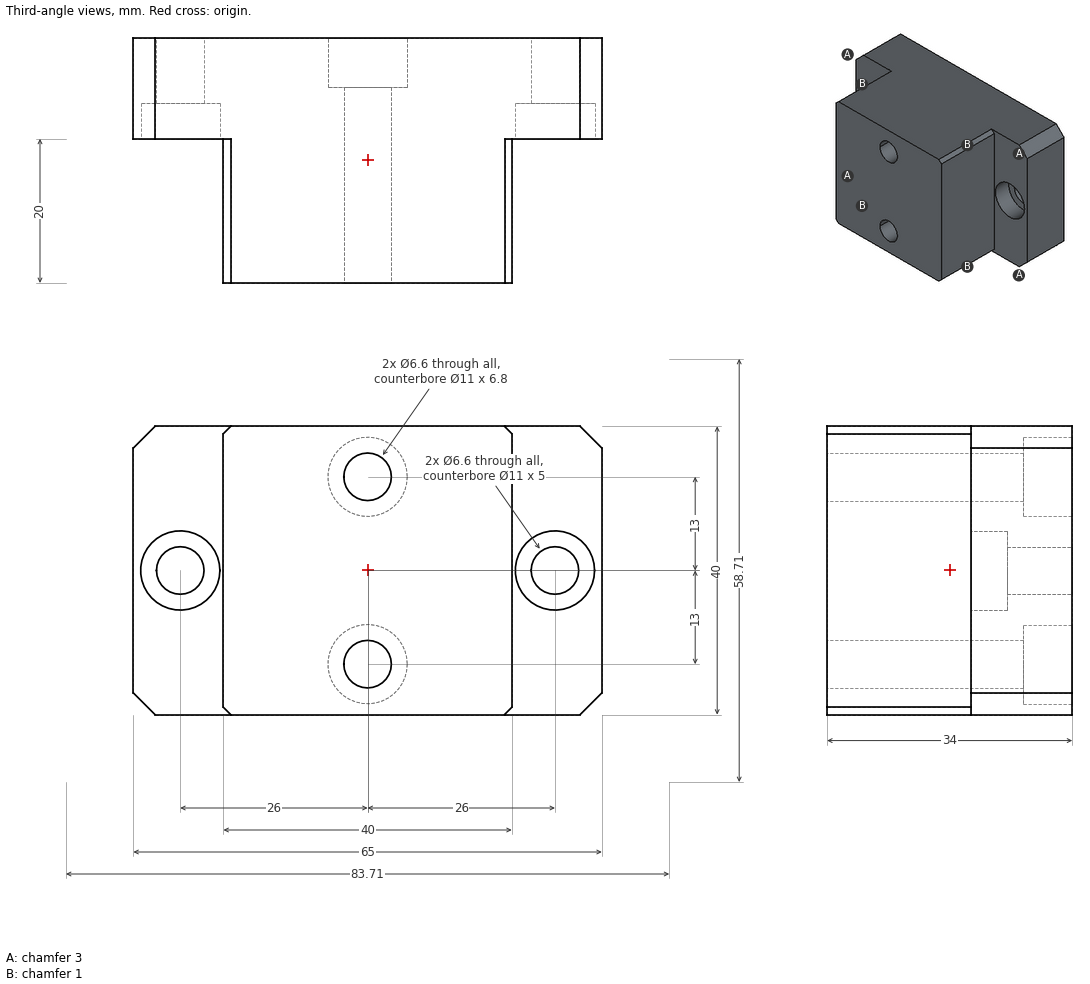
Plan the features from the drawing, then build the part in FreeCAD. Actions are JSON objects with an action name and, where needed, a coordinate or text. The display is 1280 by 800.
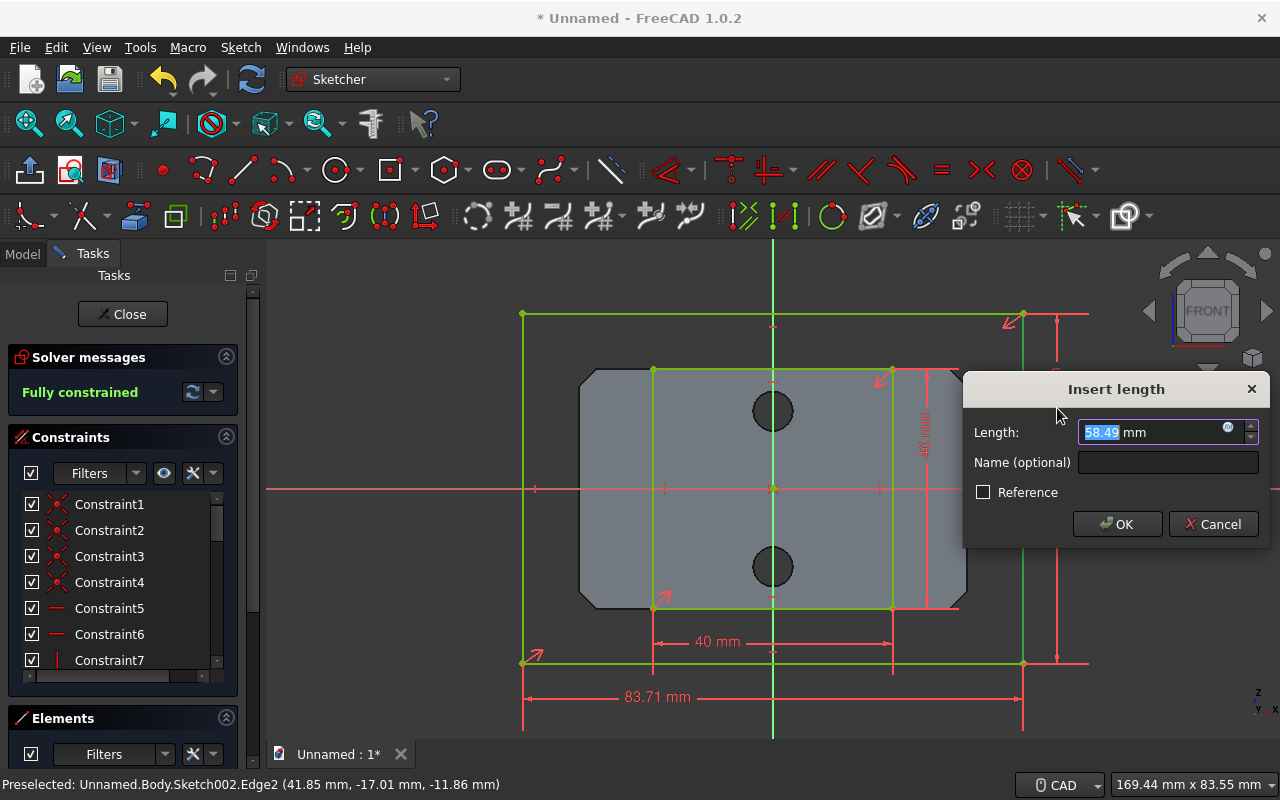
{"action": "type", "text": "58.71"}
{"action": "key", "text": "Return"}
{"action": "key", "text": "Escape"}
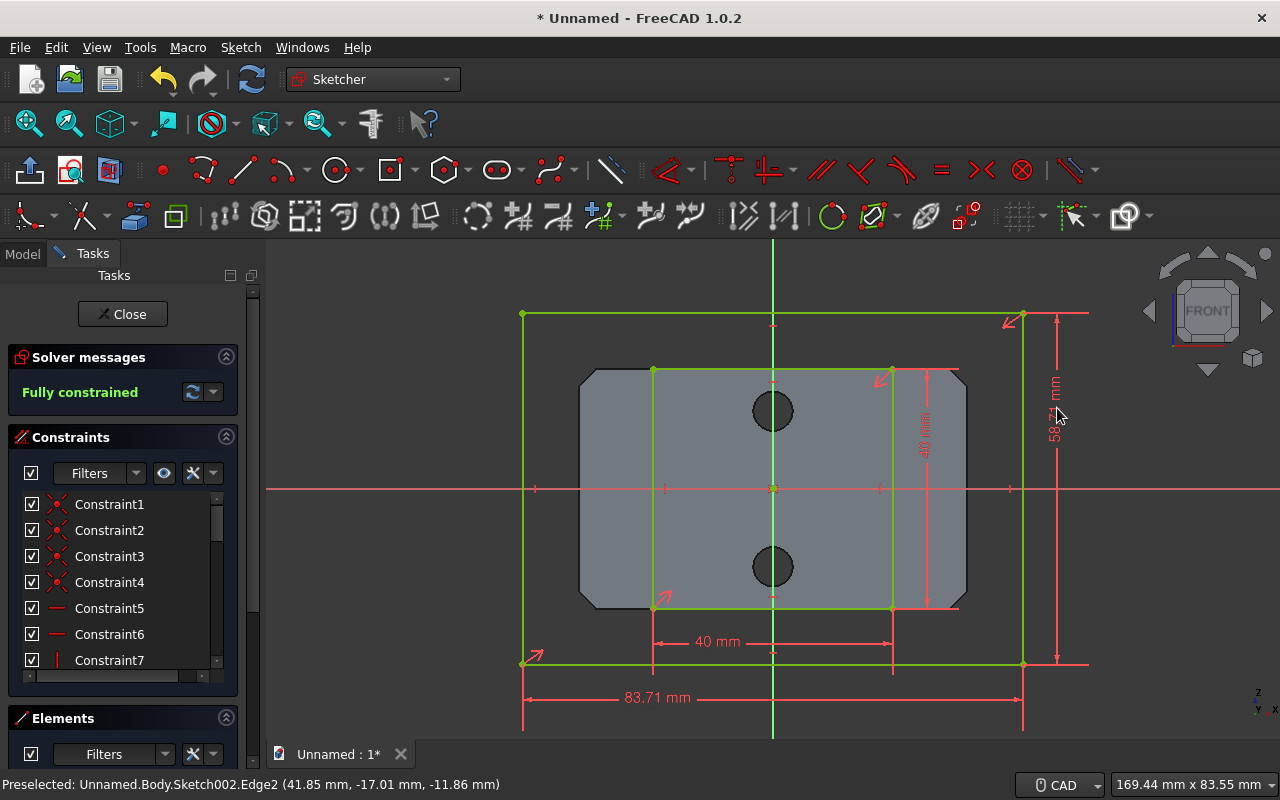
{"action": "left_click", "coordinate": [123, 314]}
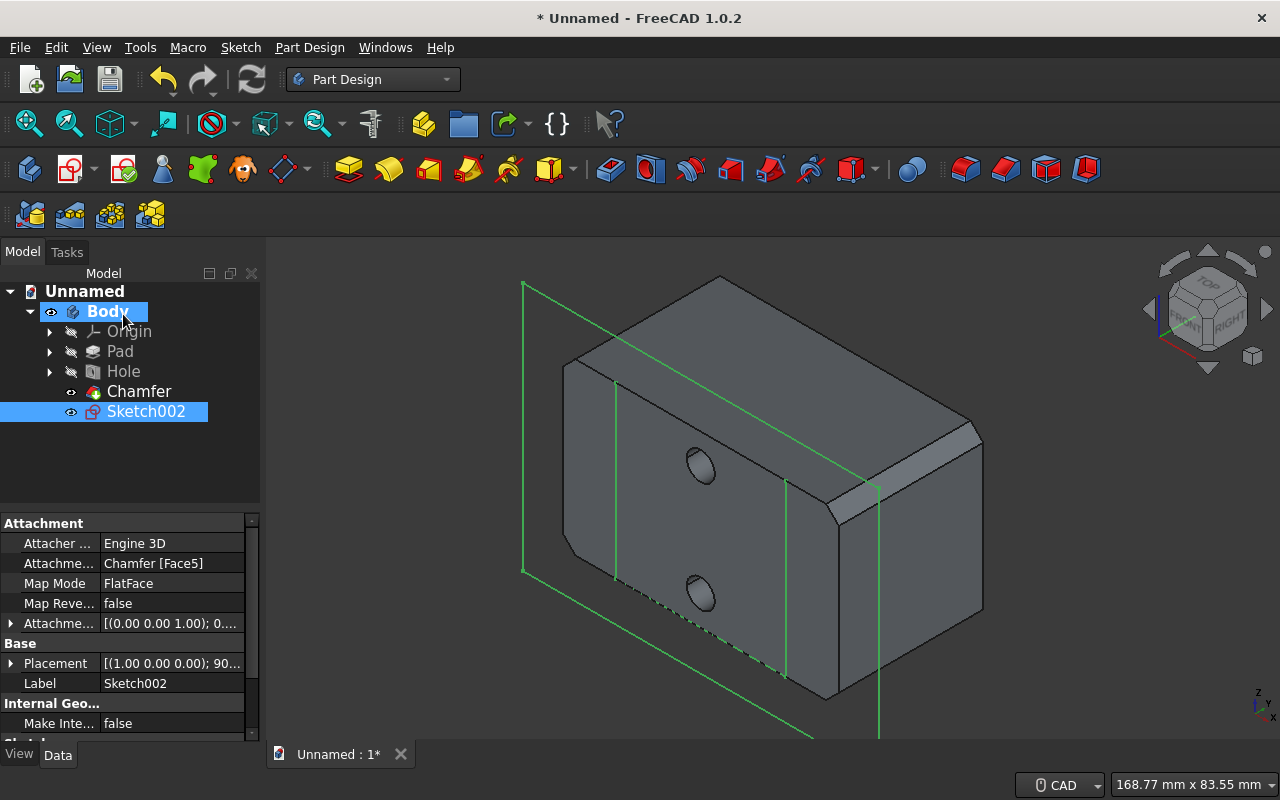
{"action": "left_click", "coordinate": [612, 170]}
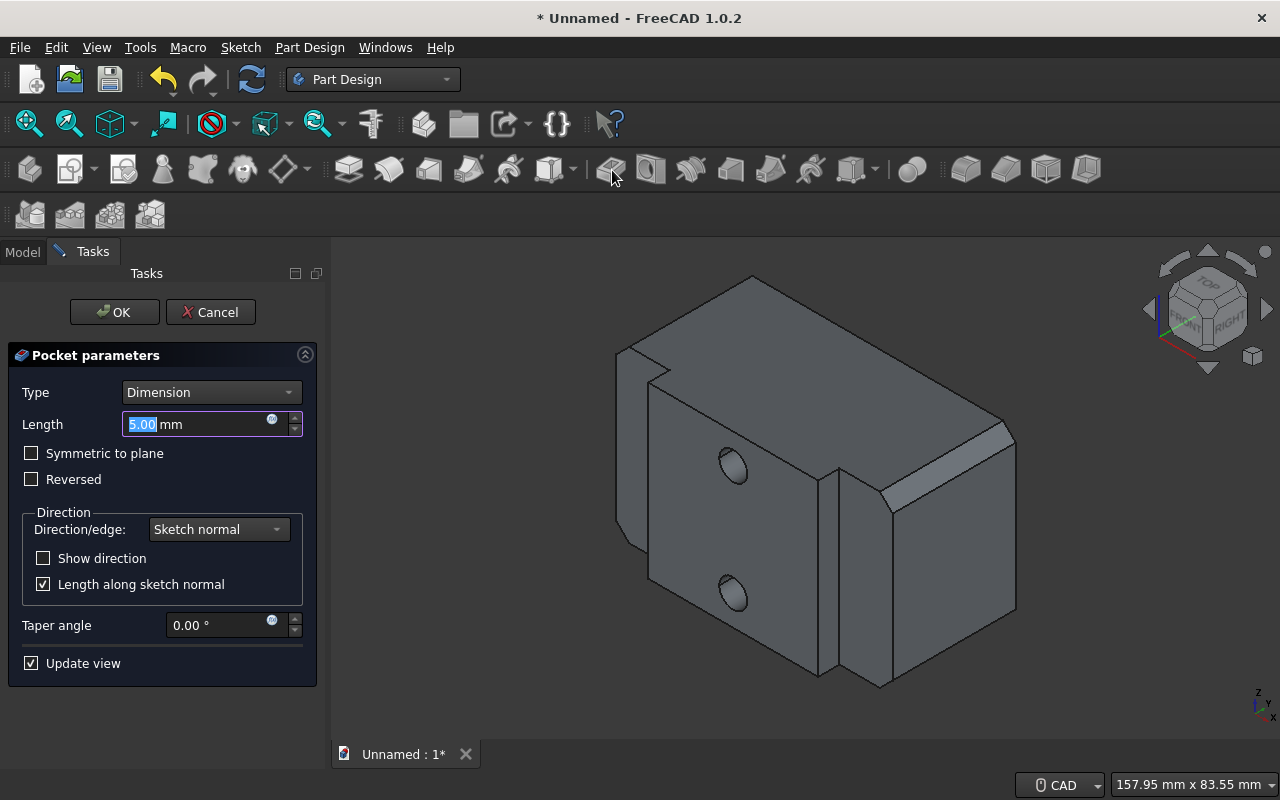
{"action": "type", "text": "20"}
{"action": "key", "text": "Tab"}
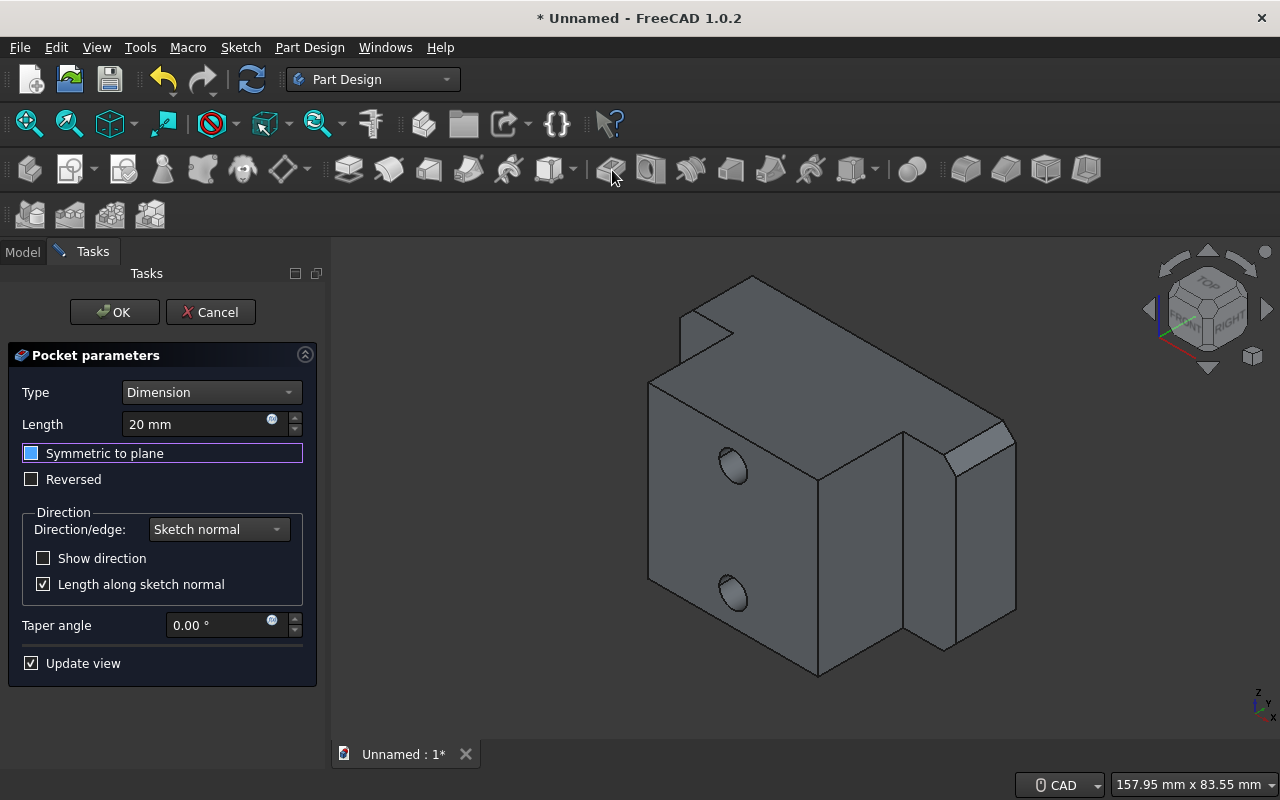
{"action": "left_click", "coordinate": [115, 312]}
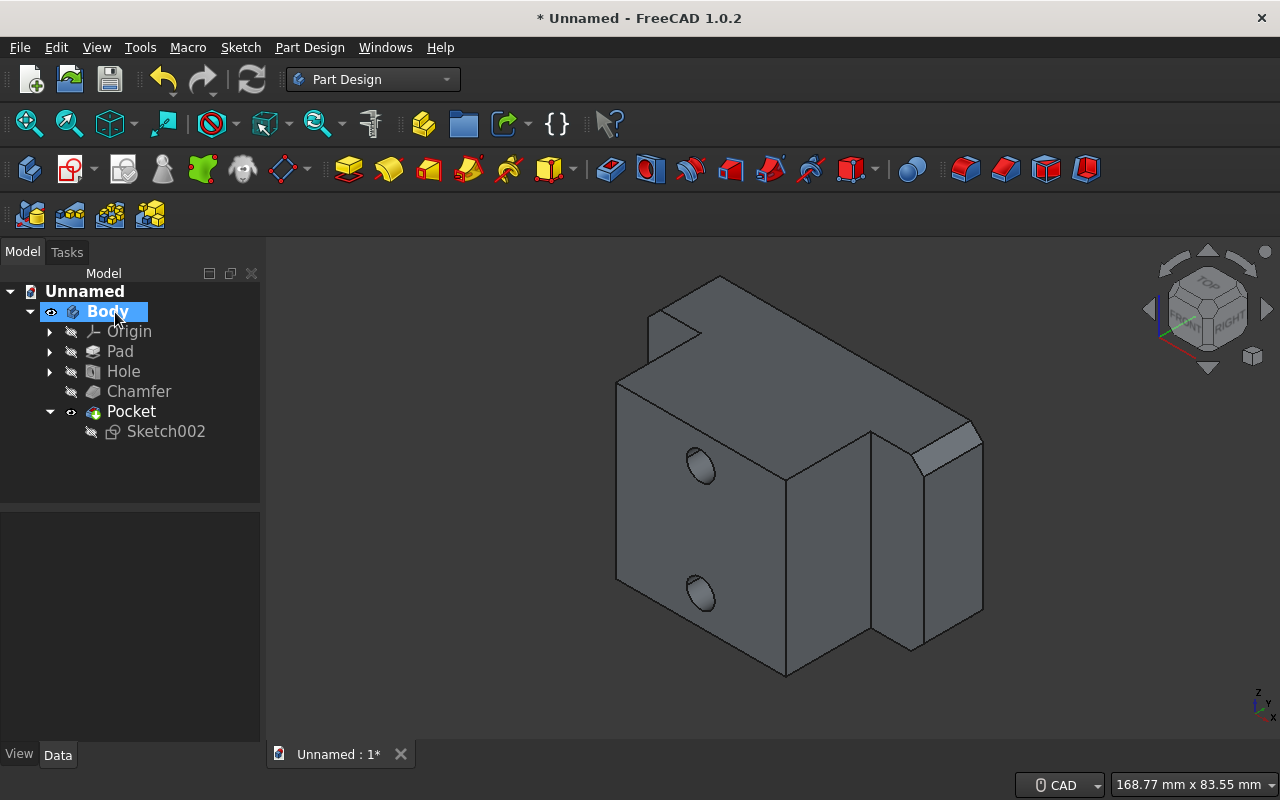
{"action": "left_click", "coordinate": [897, 488]}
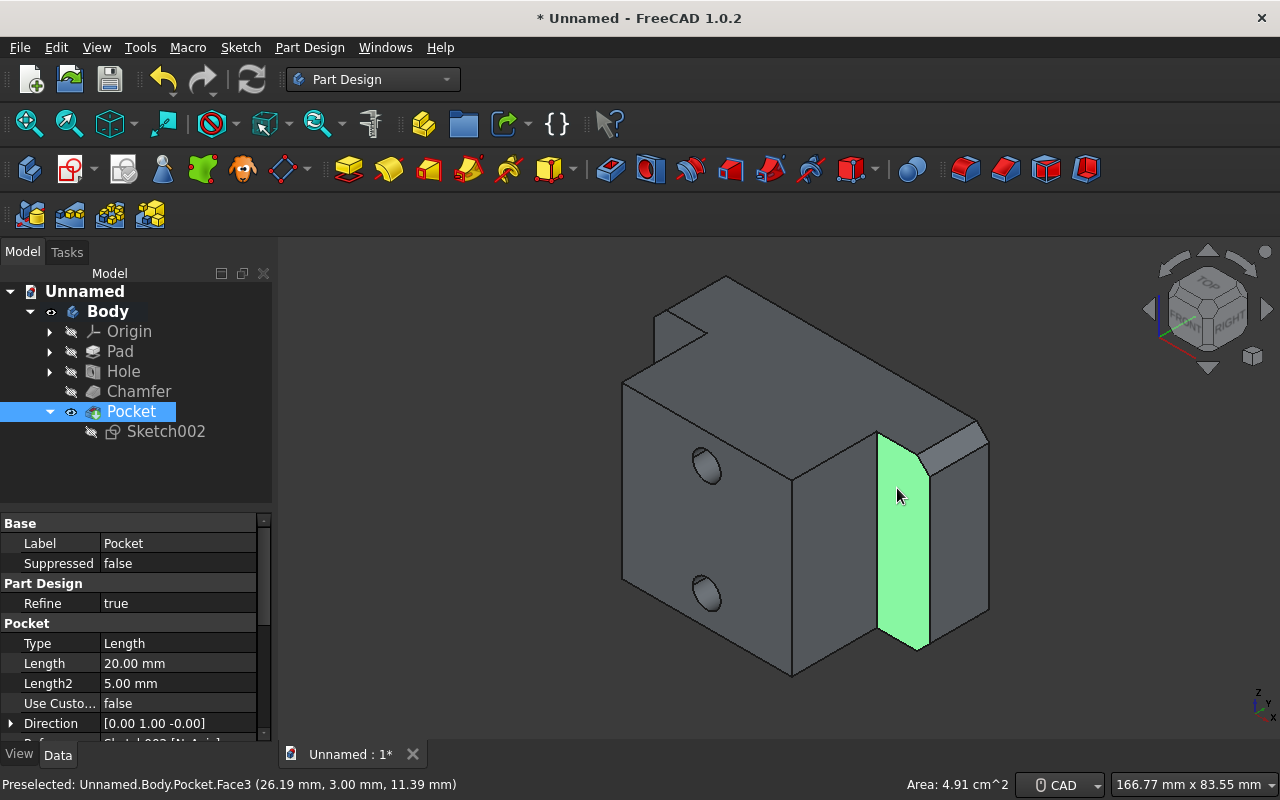
{"action": "left_click", "coordinate": [70, 170]}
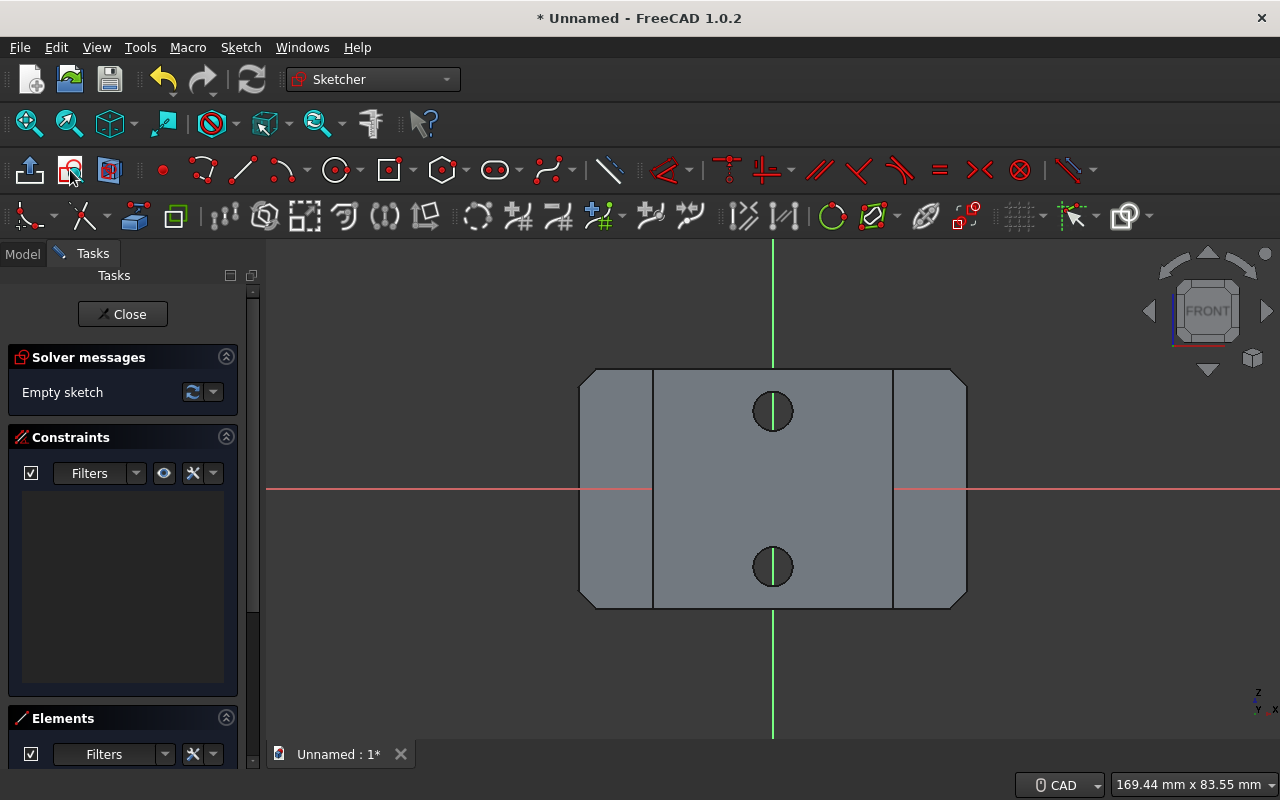
{"action": "scroll", "coordinate": [856, 489], "scroll_direction": "up", "scroll_amount": 3}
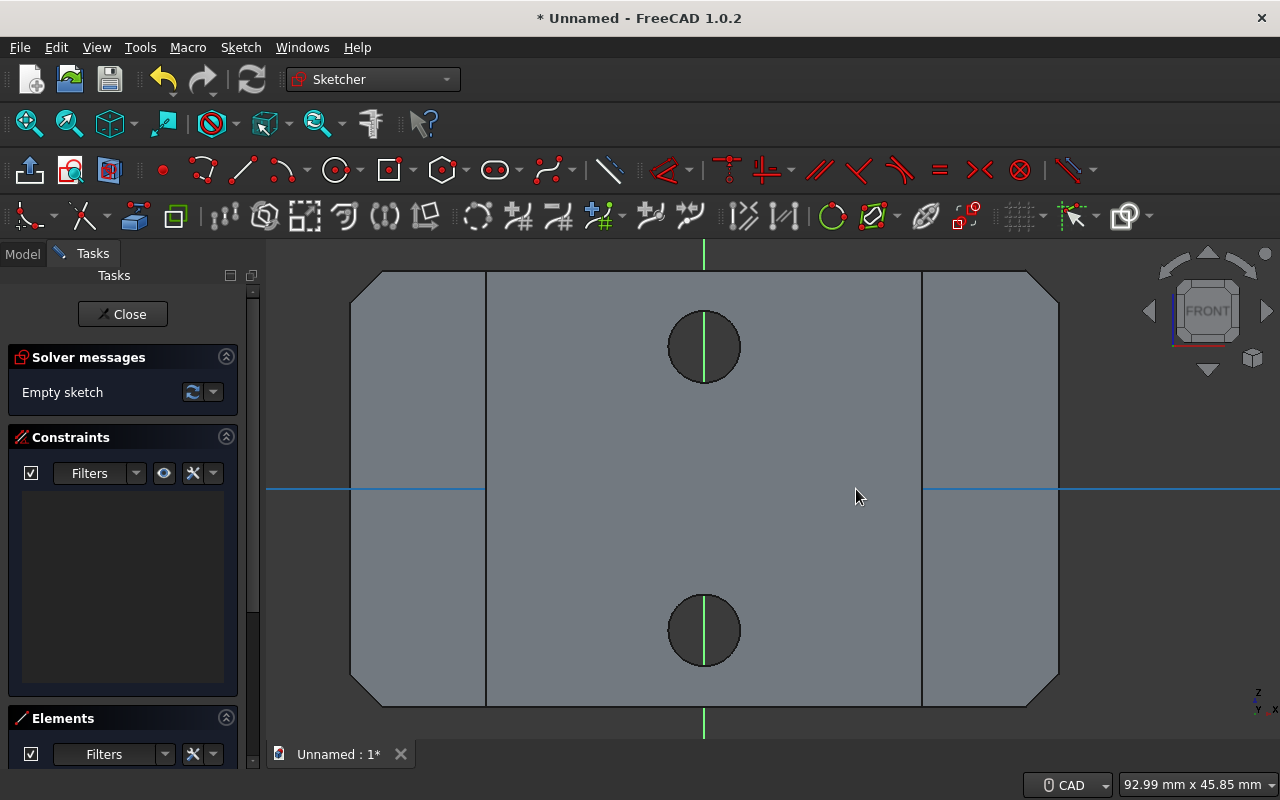
{"action": "left_click", "coordinate": [336, 170]}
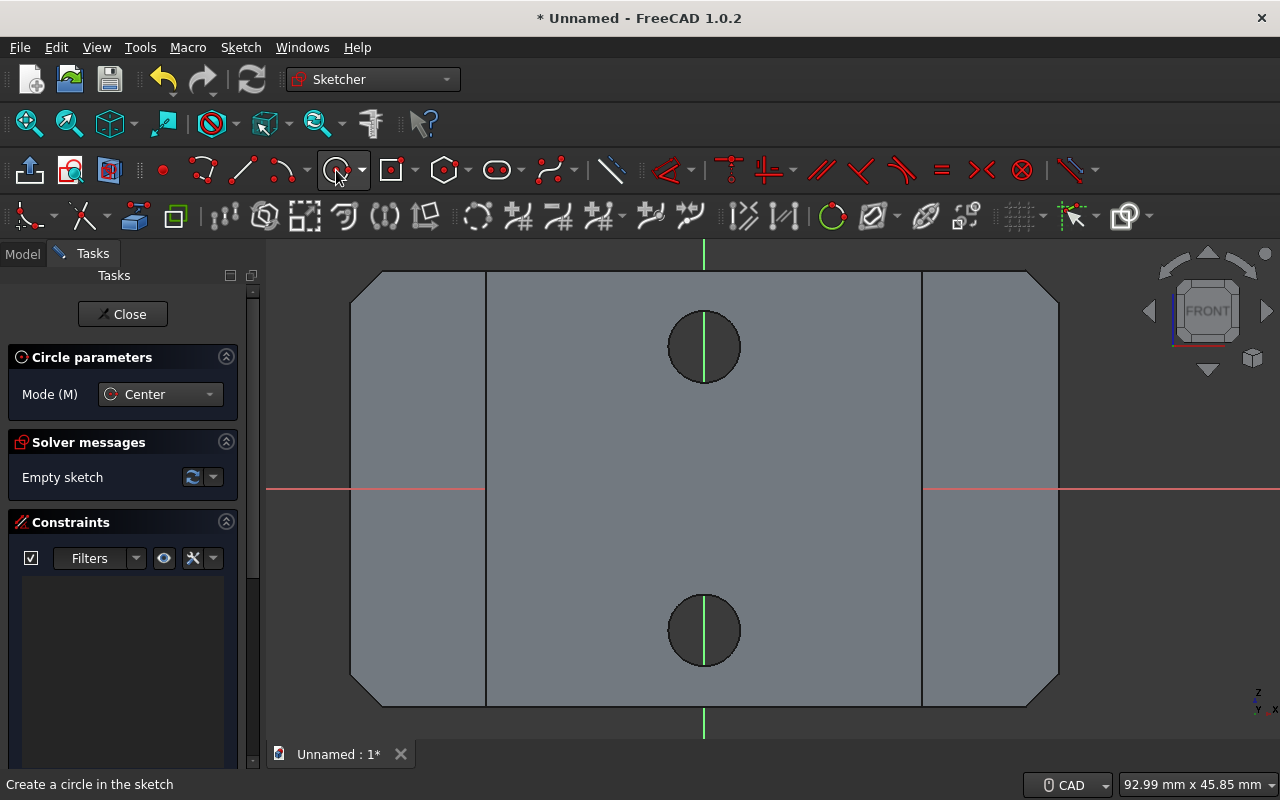
{"action": "left_click", "coordinate": [988, 489]}
{"action": "left_click", "coordinate": [1013, 463]}